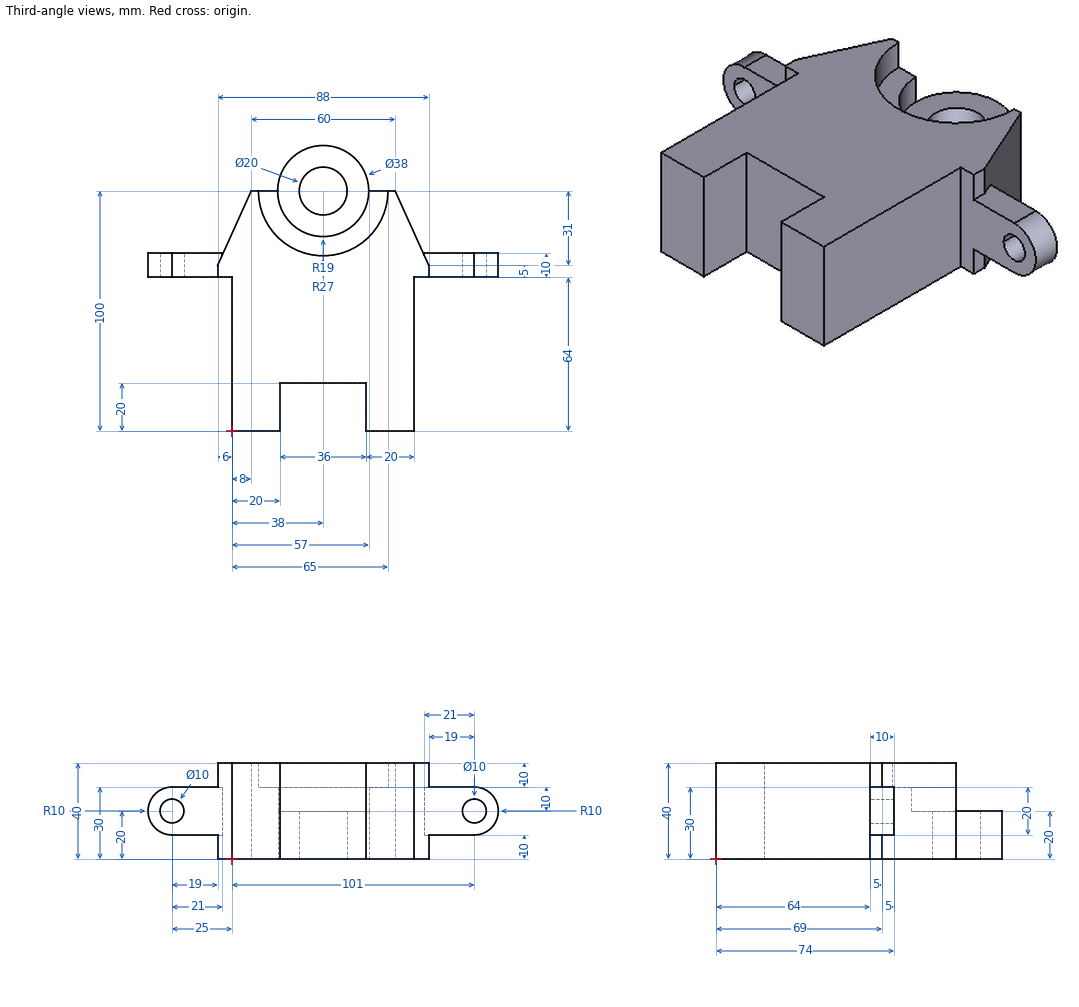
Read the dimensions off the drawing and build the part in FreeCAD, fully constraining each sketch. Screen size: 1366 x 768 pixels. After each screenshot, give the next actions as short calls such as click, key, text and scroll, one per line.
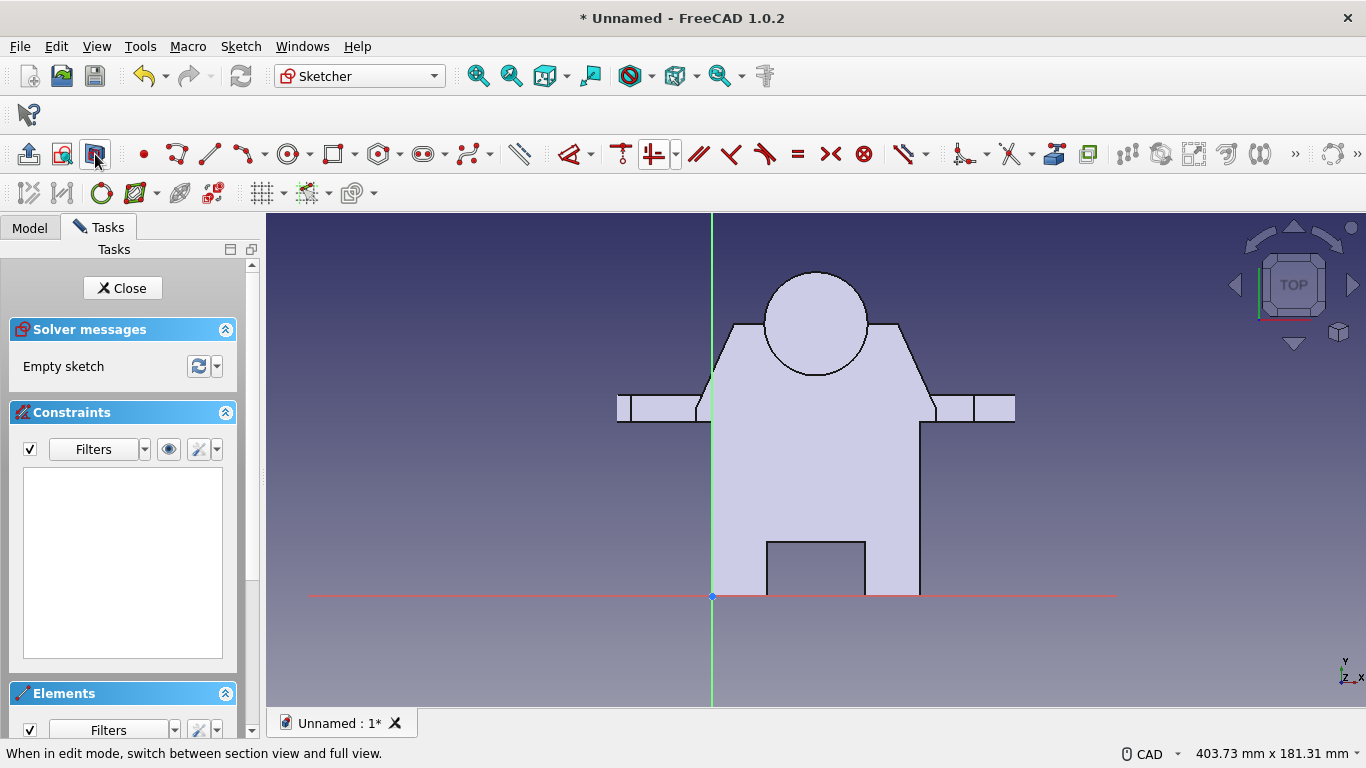
scroll(830, 297, up, 9)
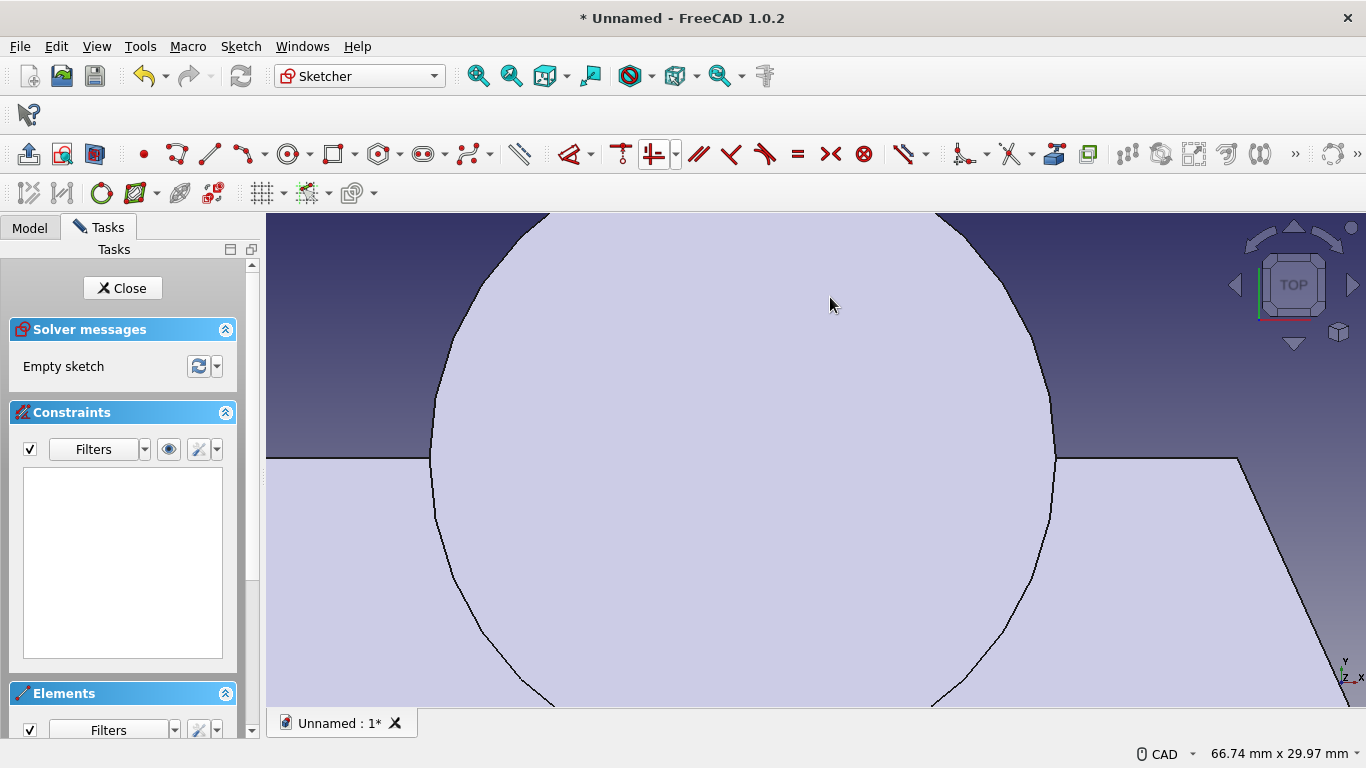
click(288, 154)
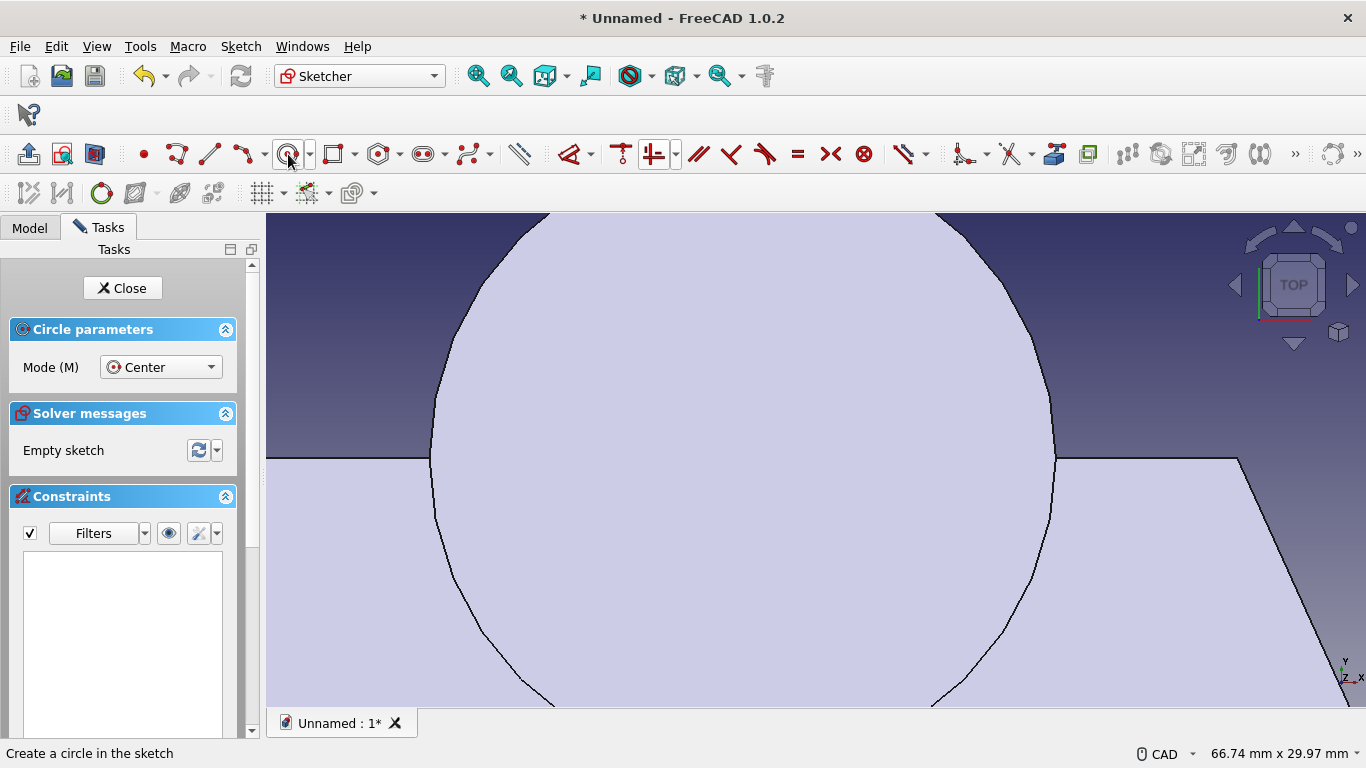
click(743, 458)
click(859, 342)
key(Escape)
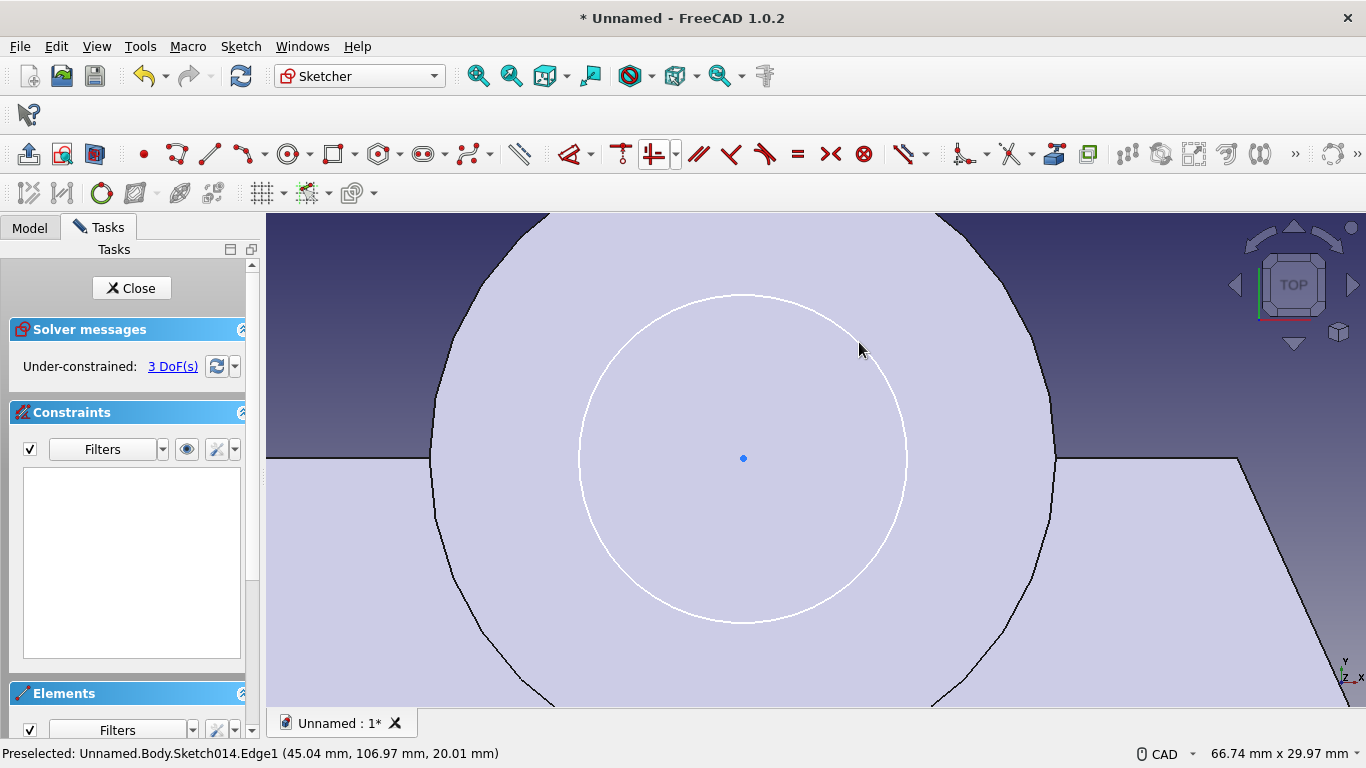
click(568, 154)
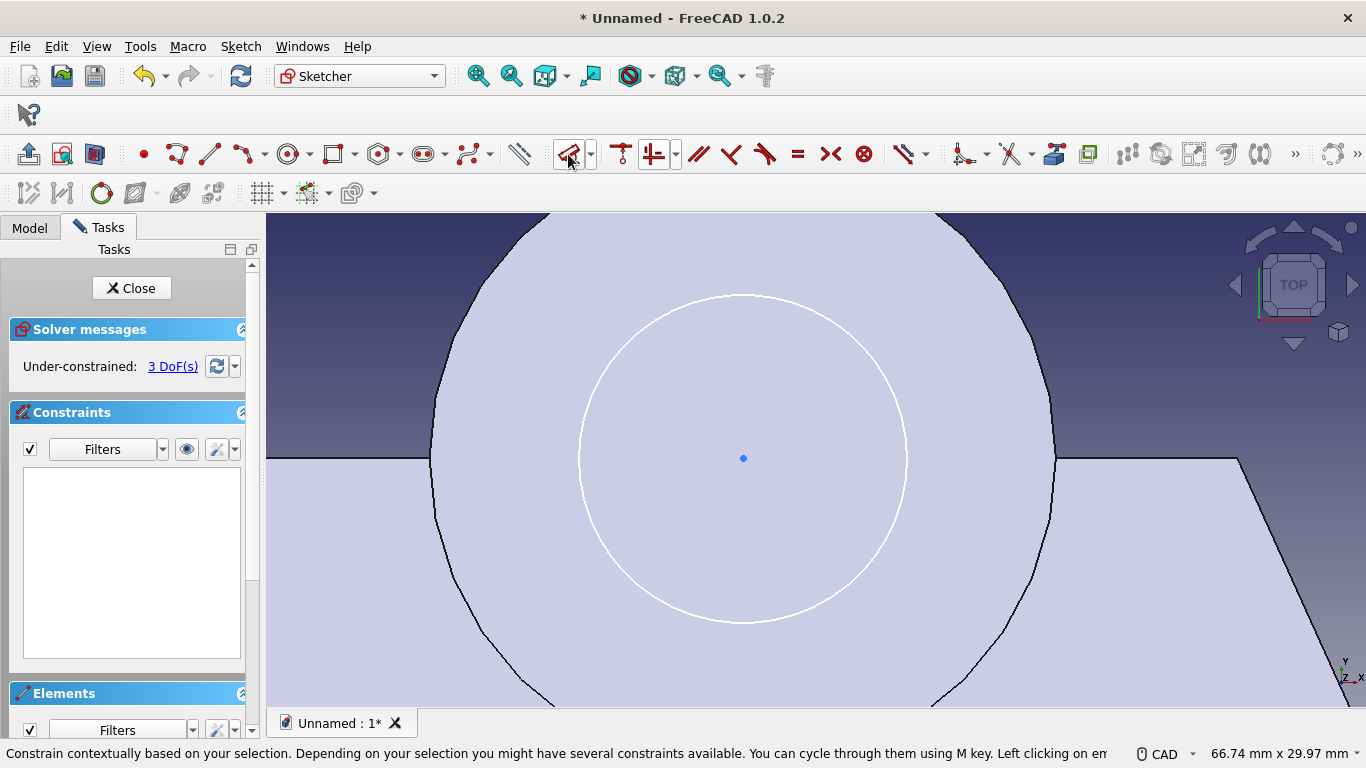
click(859, 343)
click(882, 320)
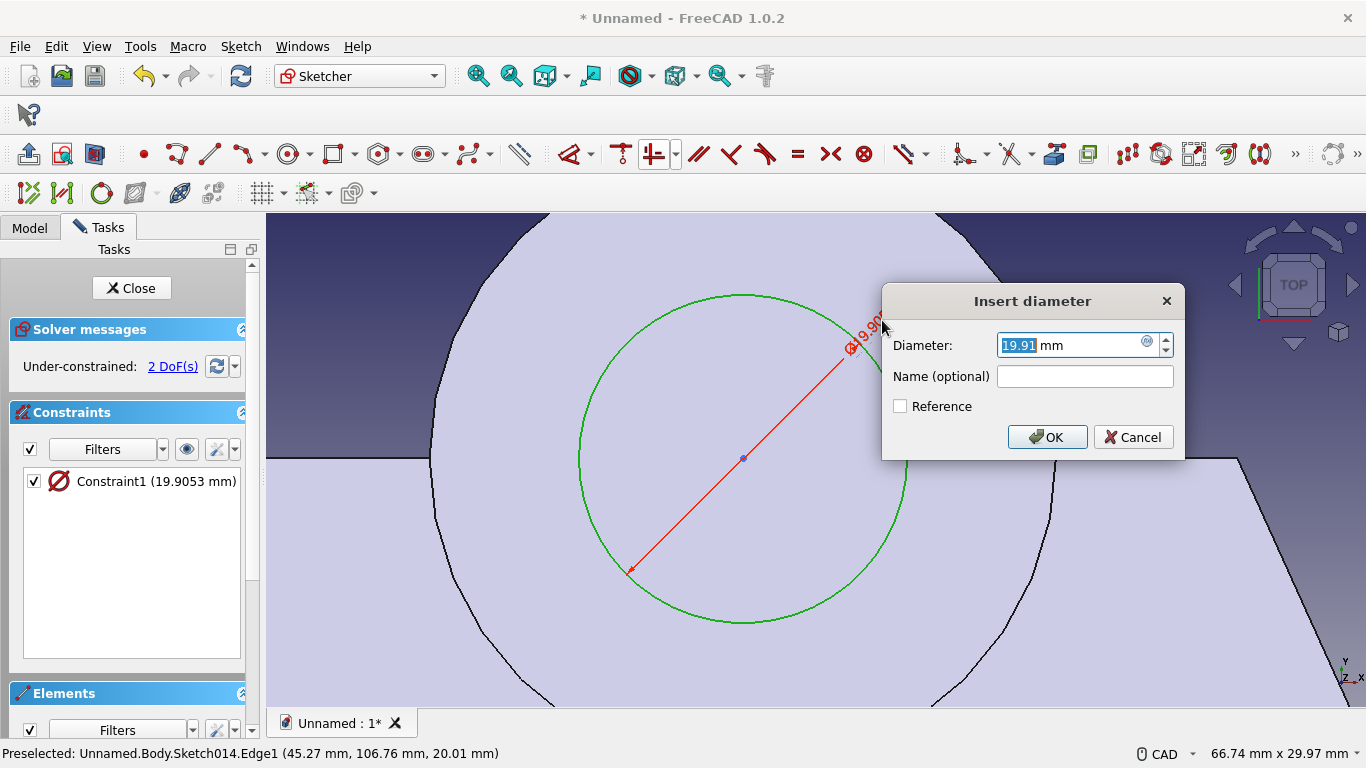
text(20)
key(Return)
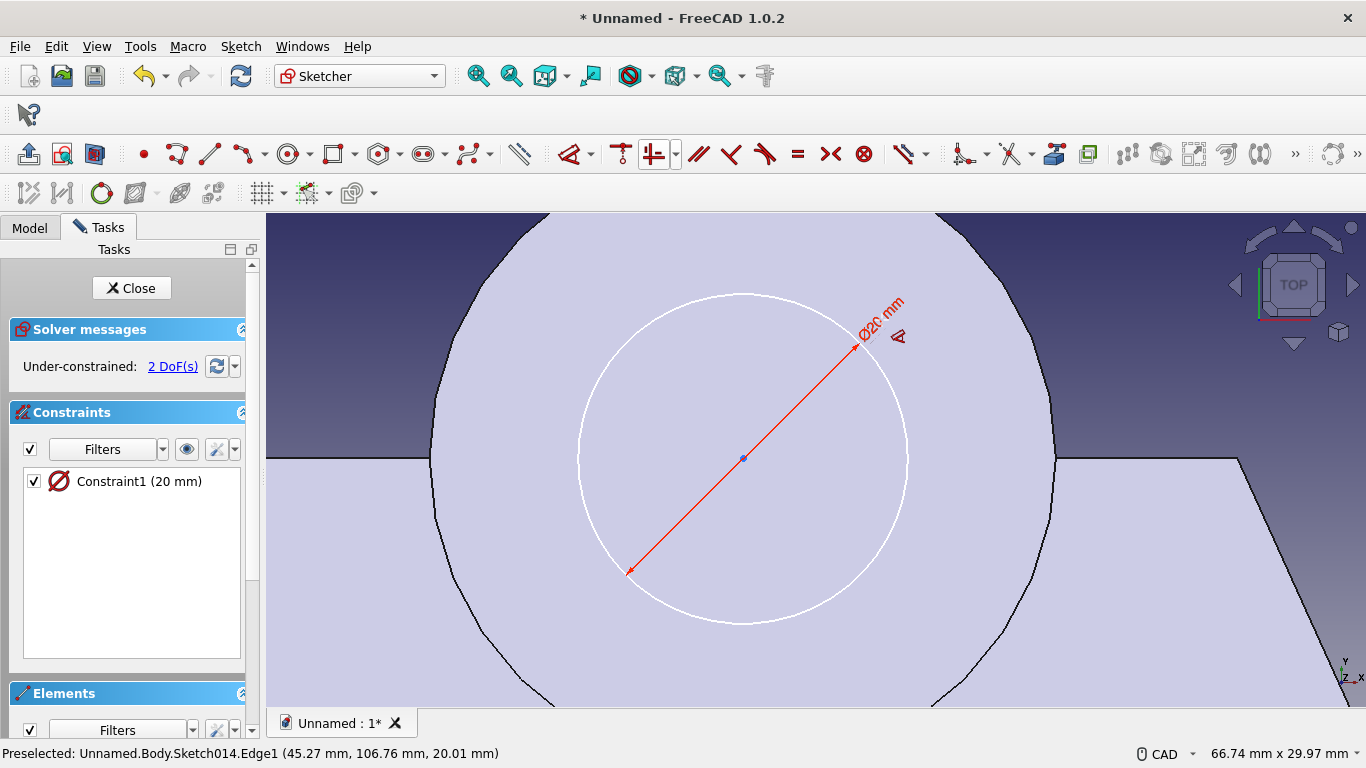
click(743, 459)
click(518, 425)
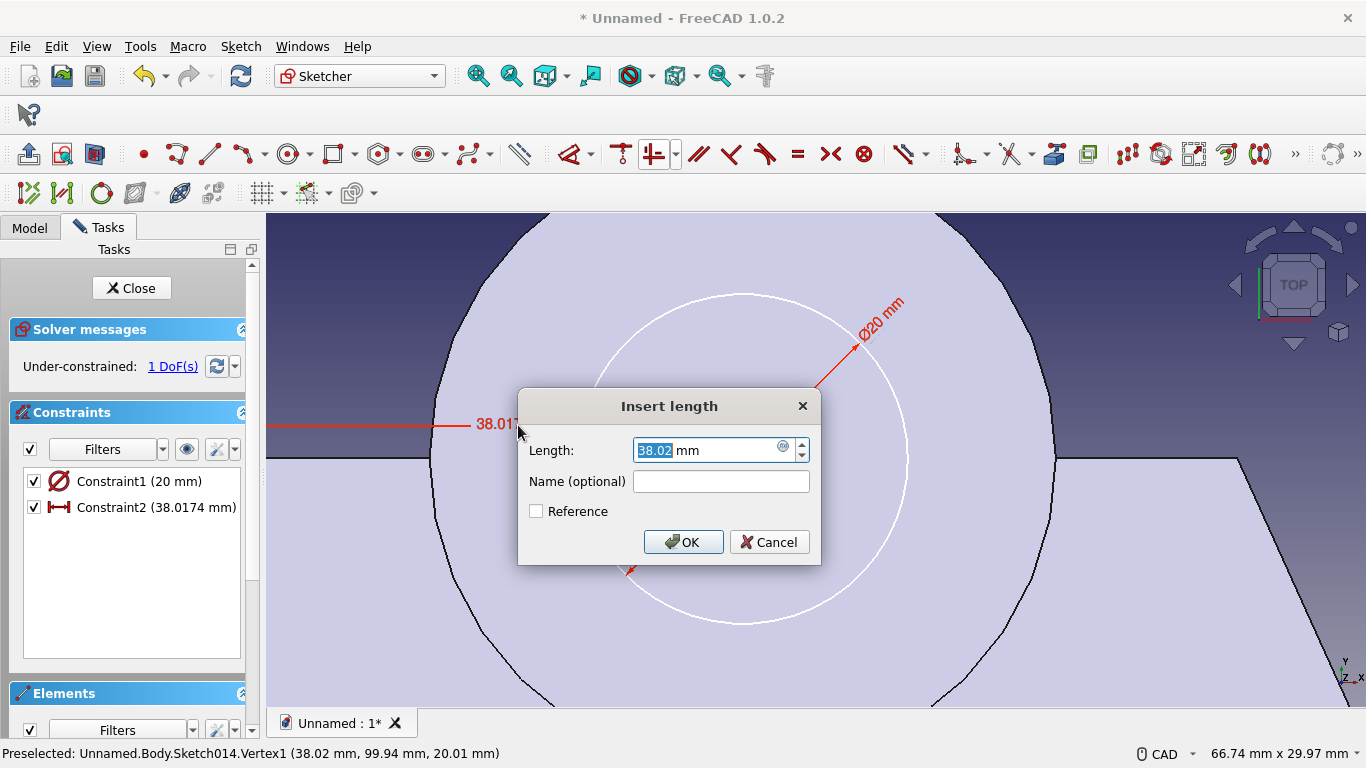
text(38)
key(Return)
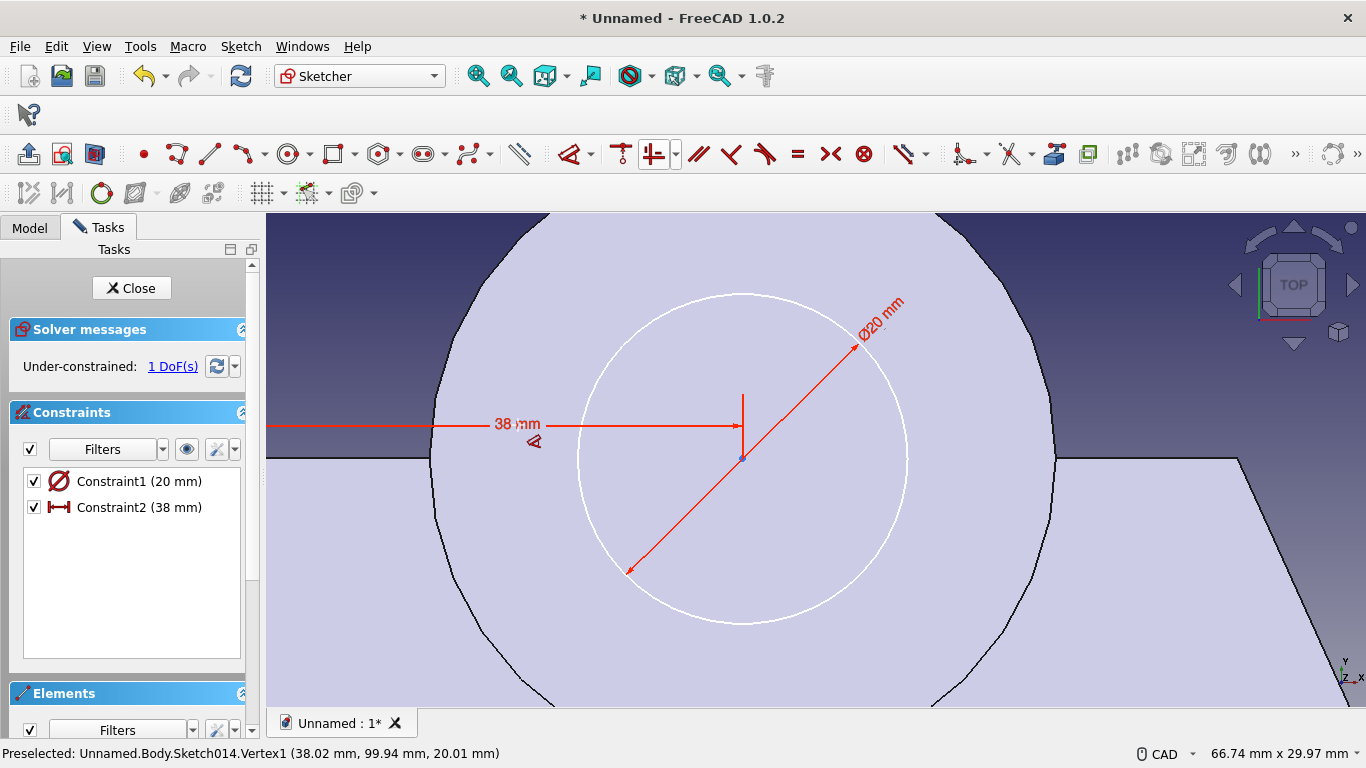
click(743, 459)
click(777, 569)